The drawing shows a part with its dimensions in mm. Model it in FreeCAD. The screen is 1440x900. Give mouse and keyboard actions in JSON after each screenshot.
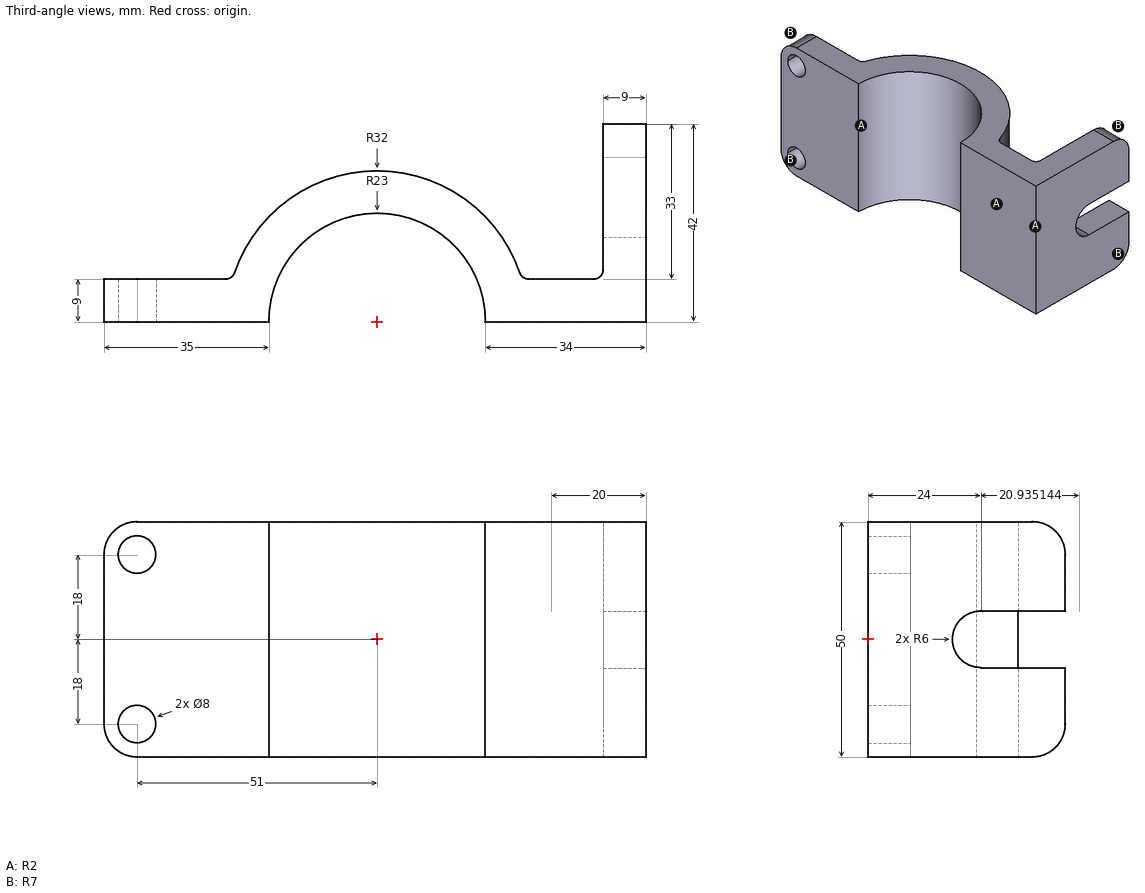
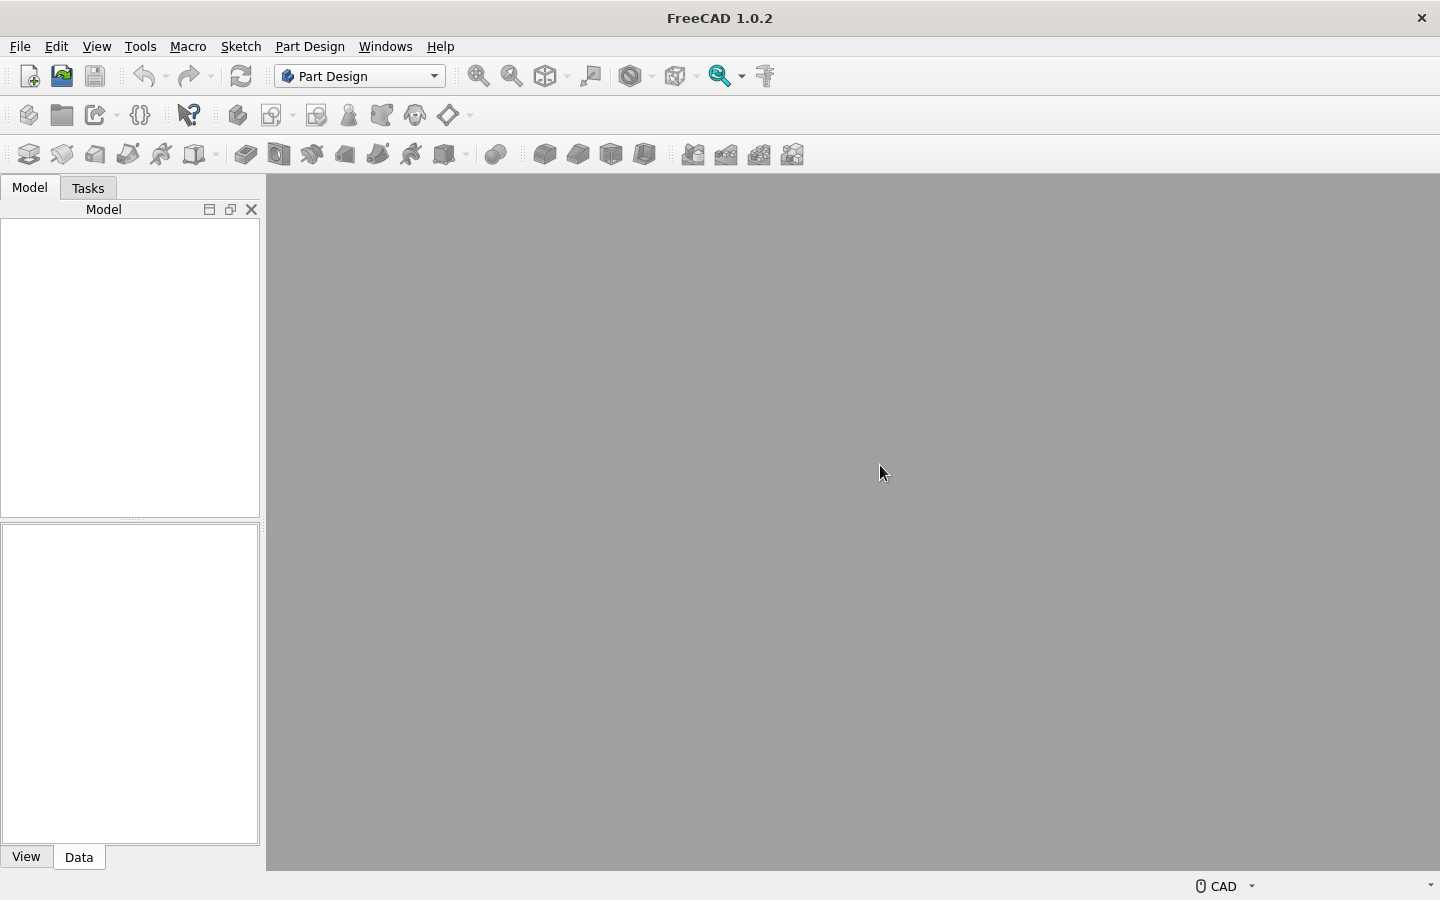
{"action": "left_click", "coordinate": [29, 76]}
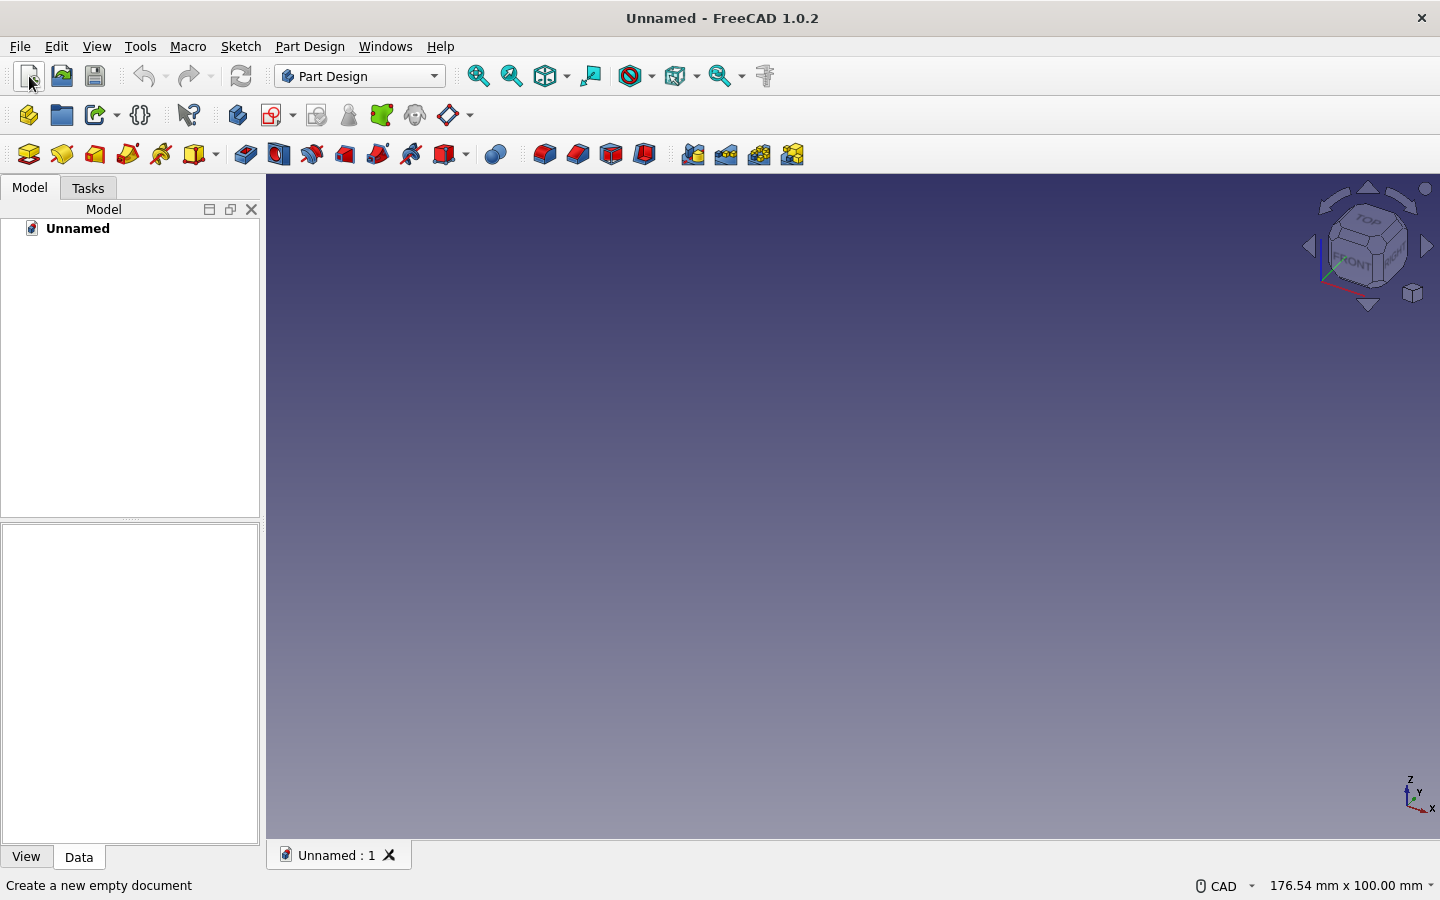
{"action": "left_click", "coordinate": [270, 116]}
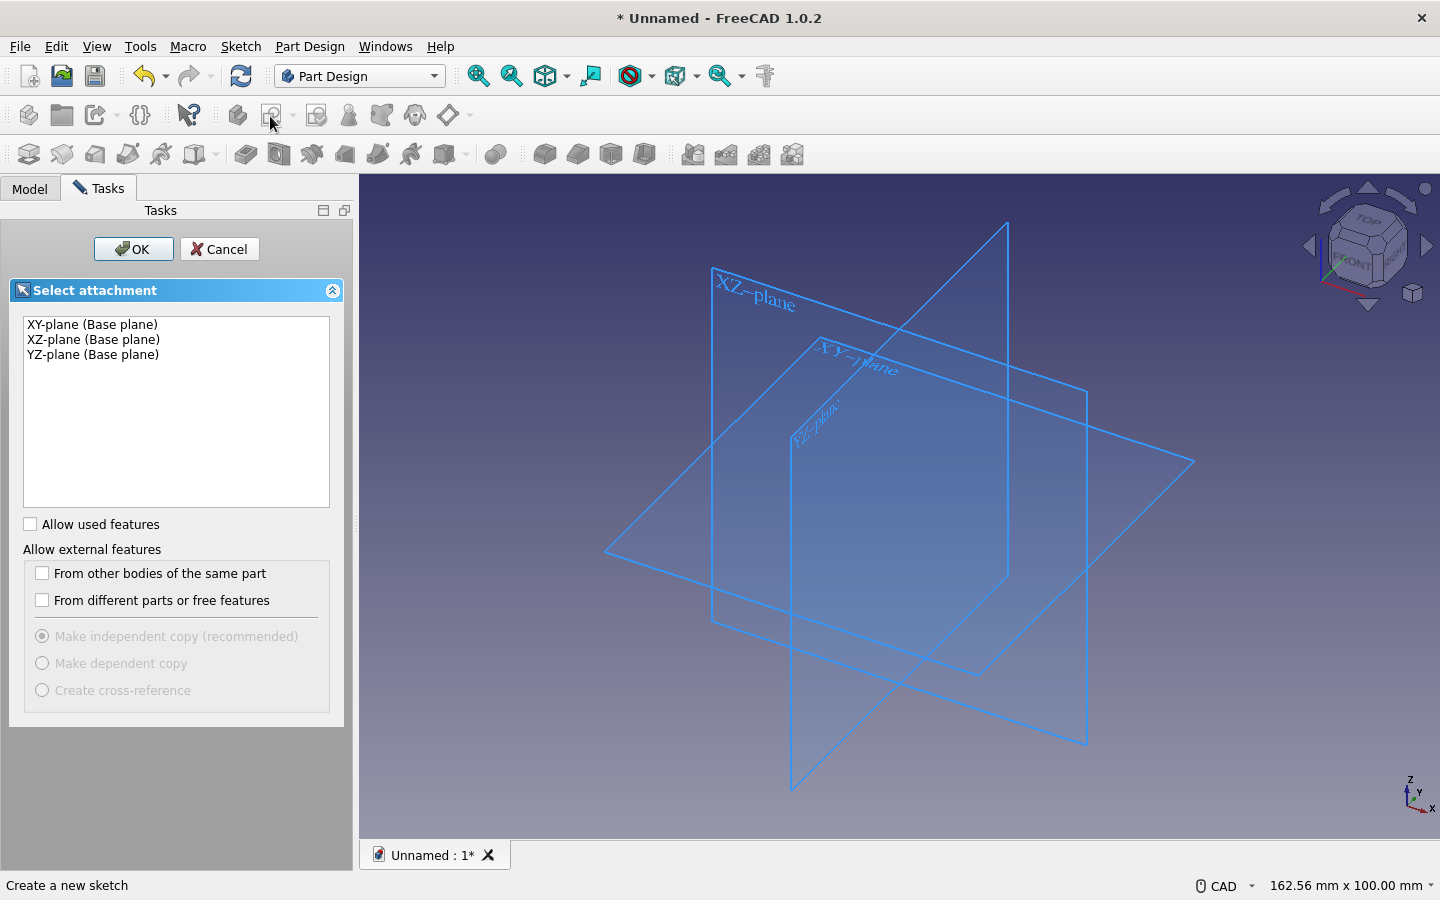
{"action": "left_click", "coordinate": [84, 324]}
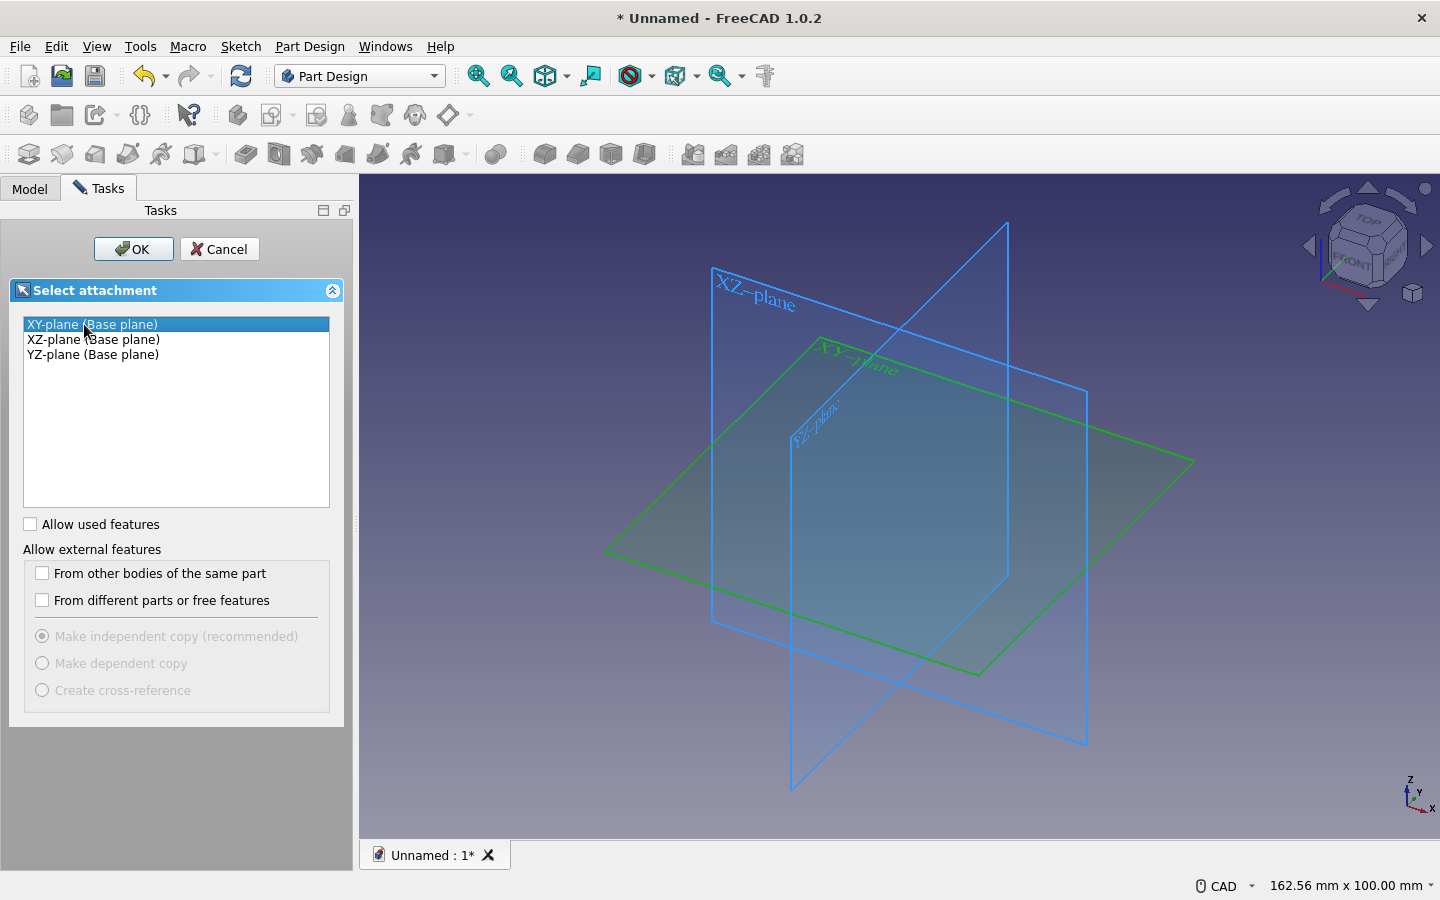
{"action": "left_click", "coordinate": [134, 249]}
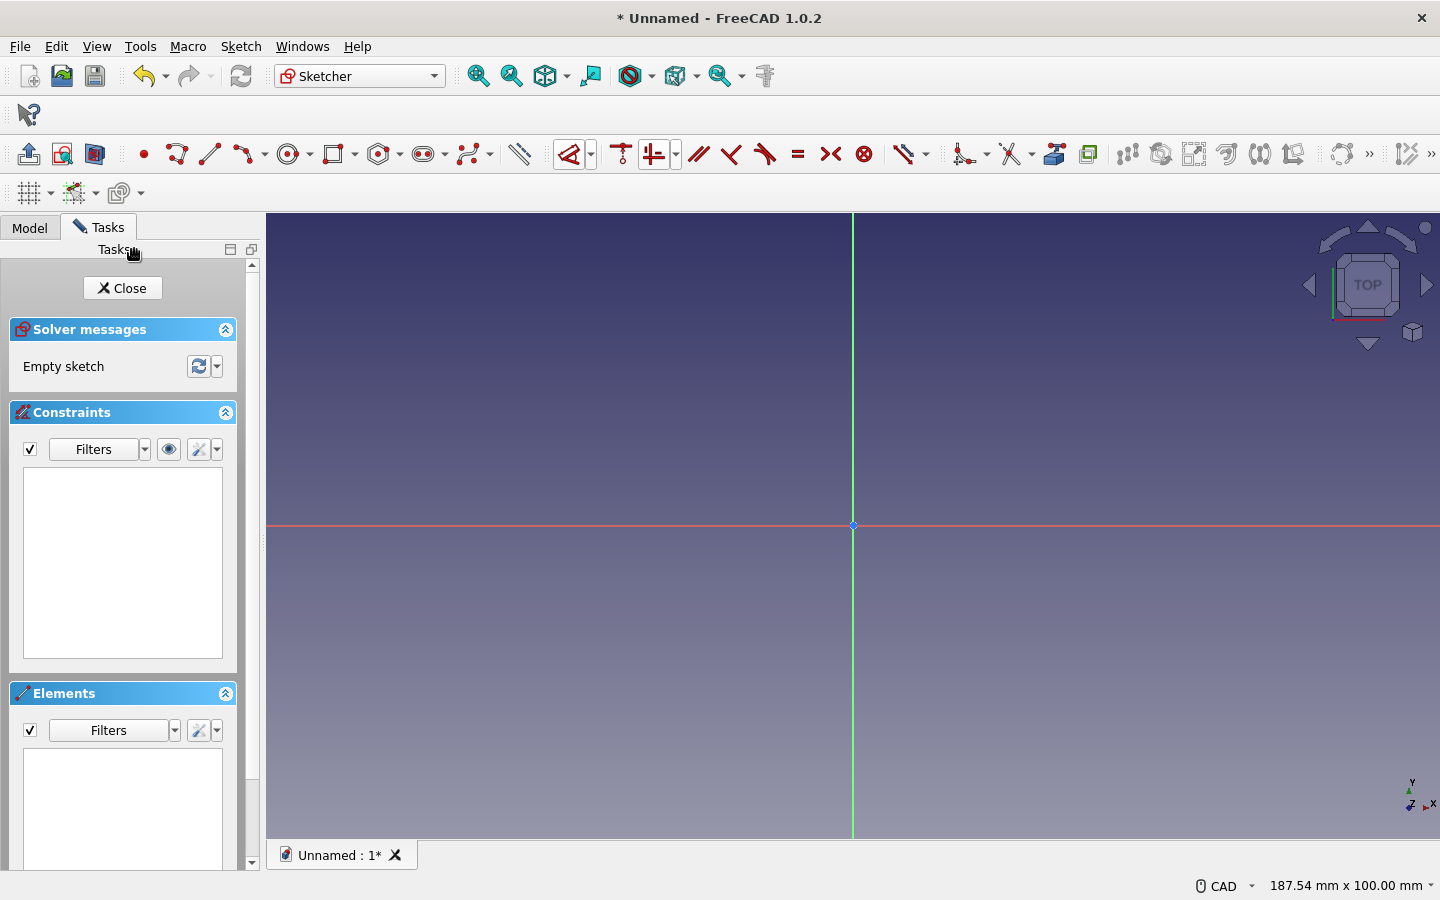
{"action": "scroll", "coordinate": [489, 811], "scroll_direction": "down", "scroll_amount": 1}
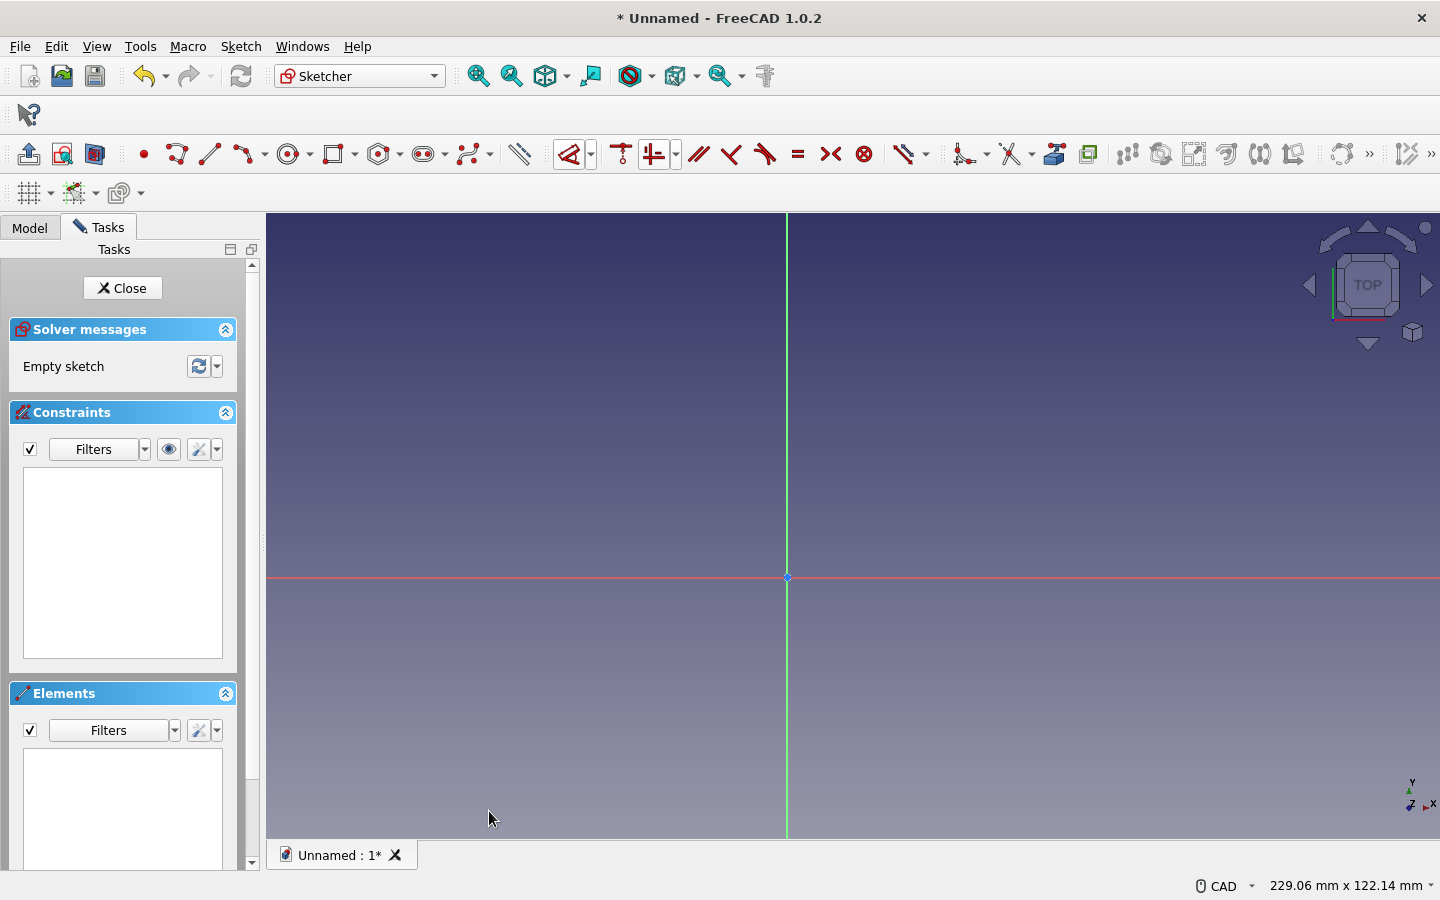
{"action": "left_click", "coordinate": [177, 154]}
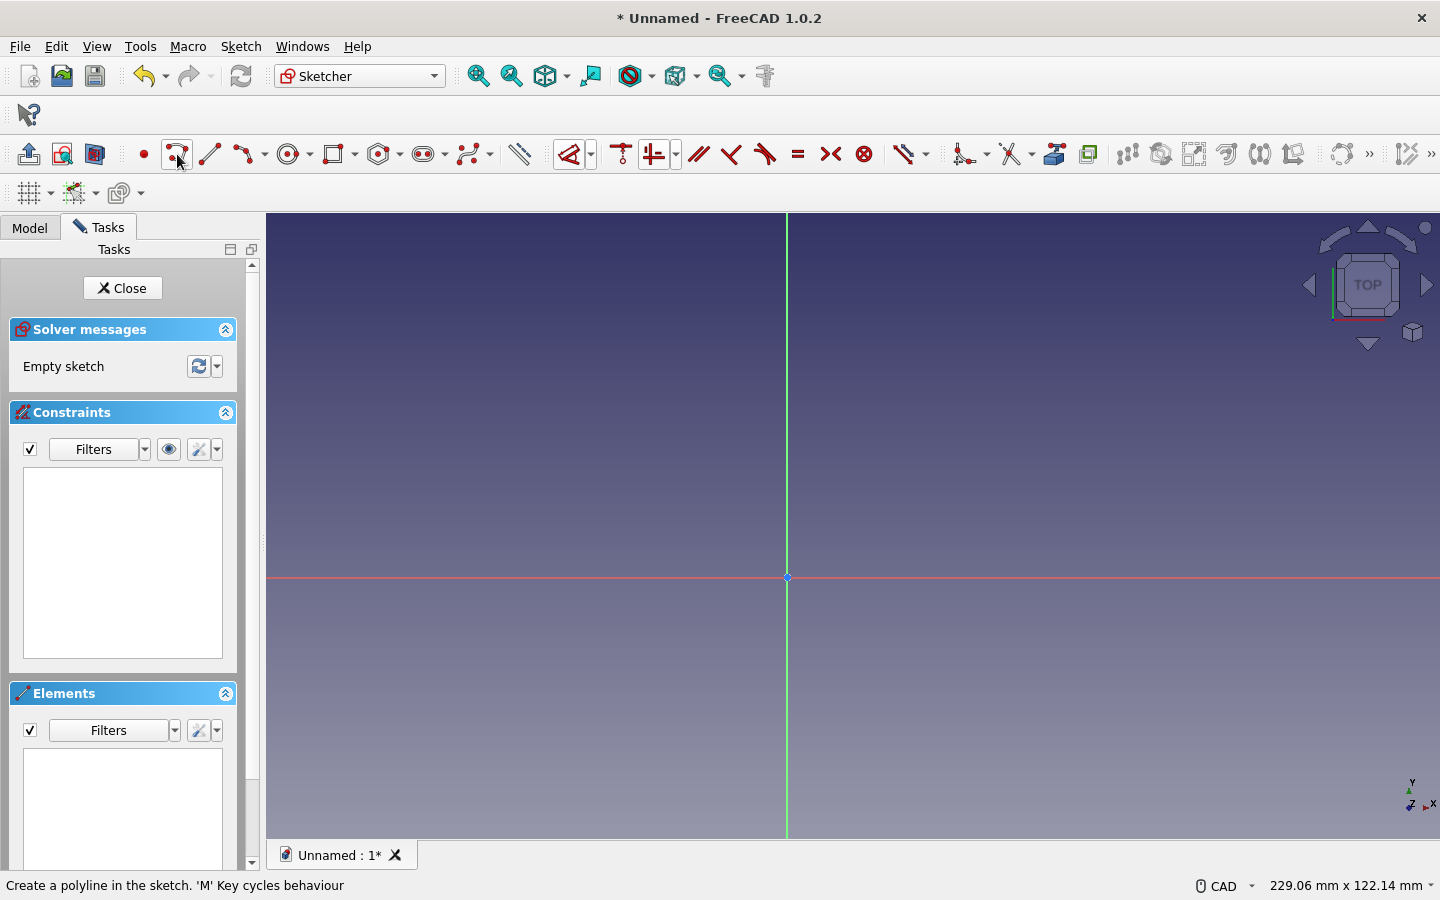
{"action": "left_click", "coordinate": [905, 578]}
{"action": "left_click", "coordinate": [1079, 569]}
{"action": "left_click", "coordinate": [1079, 363]}
{"action": "left_click", "coordinate": [1033, 363]}
{"action": "left_click", "coordinate": [1033, 532]}
{"action": "left_click", "coordinate": [944, 532]}
{"action": "right_click", "coordinate": [944, 532]}